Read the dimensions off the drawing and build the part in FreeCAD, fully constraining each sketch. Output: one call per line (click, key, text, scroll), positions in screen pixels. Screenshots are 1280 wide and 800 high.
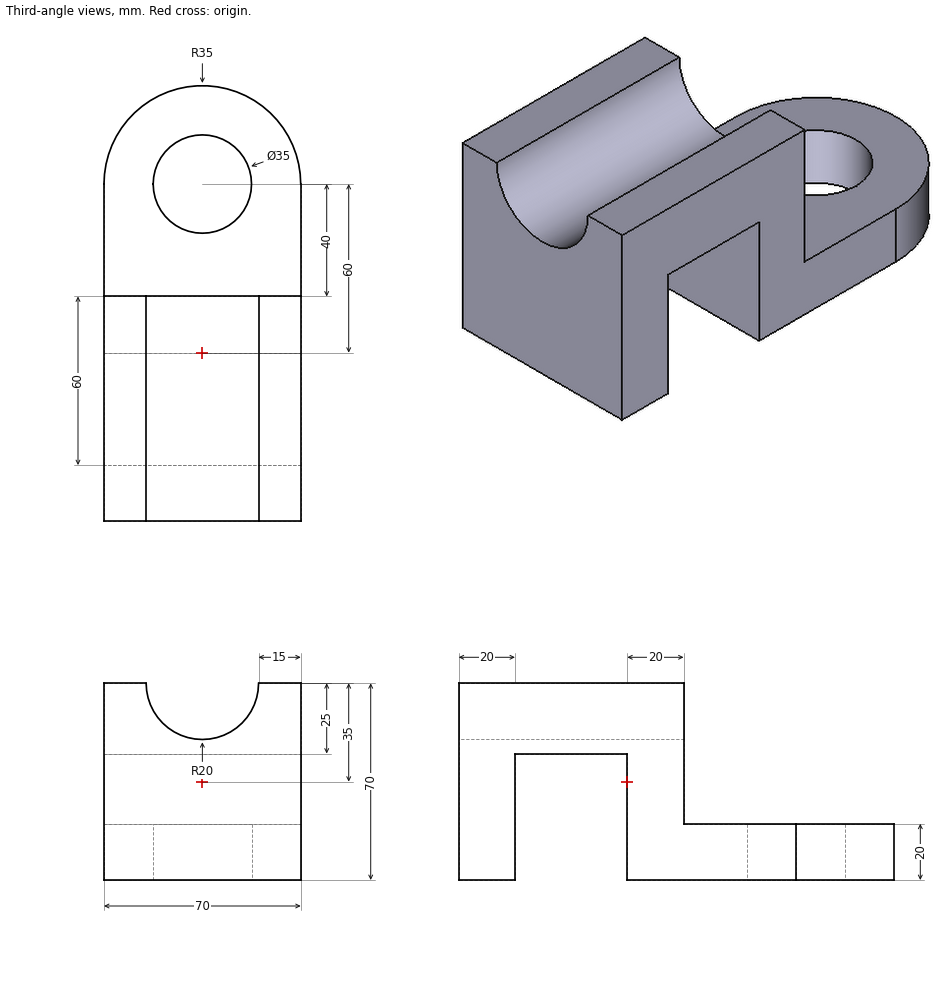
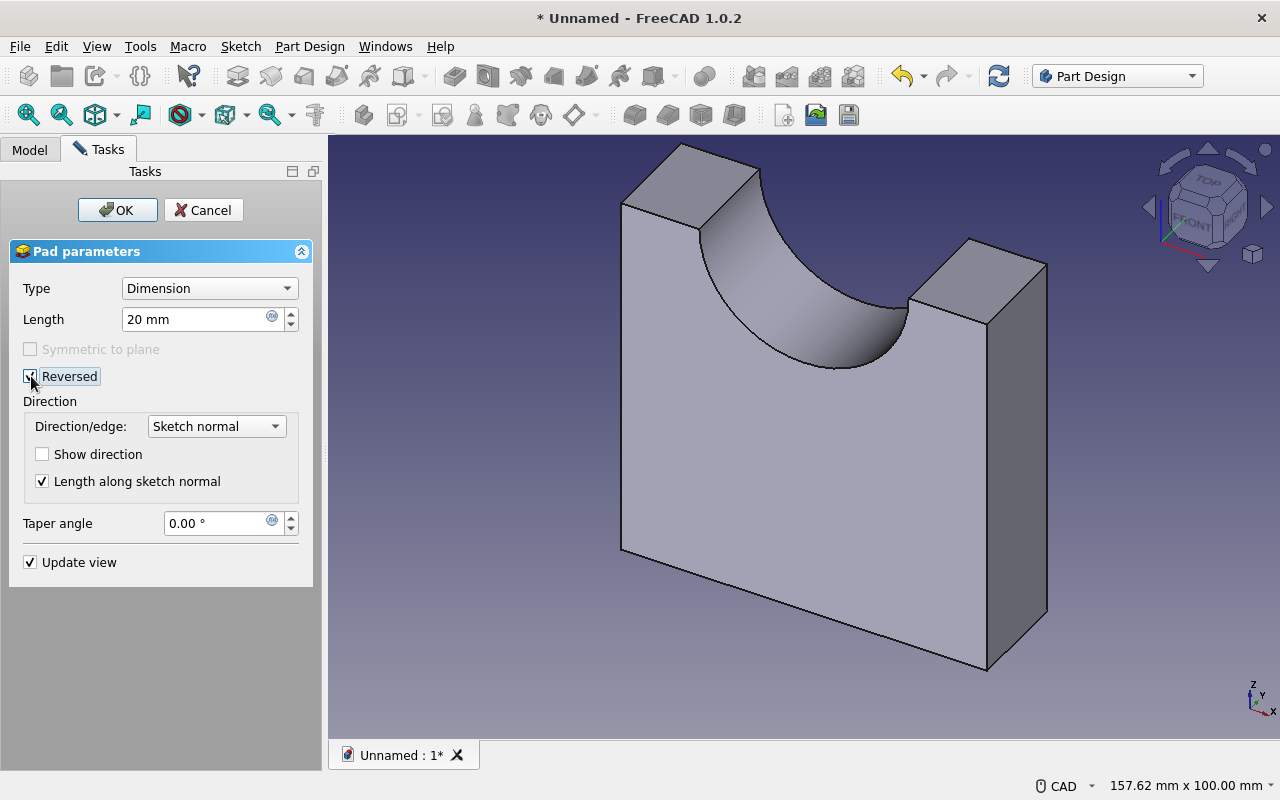
click(118, 210)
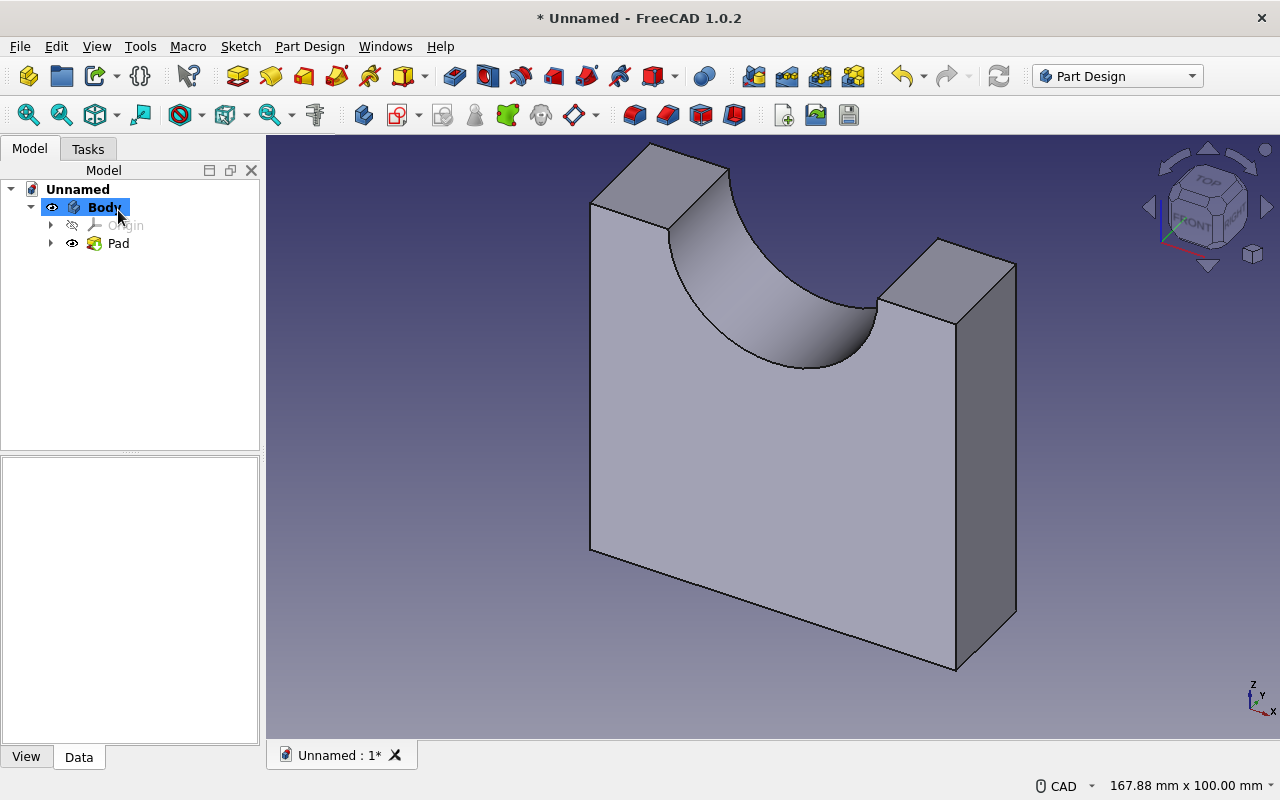
click(51, 225)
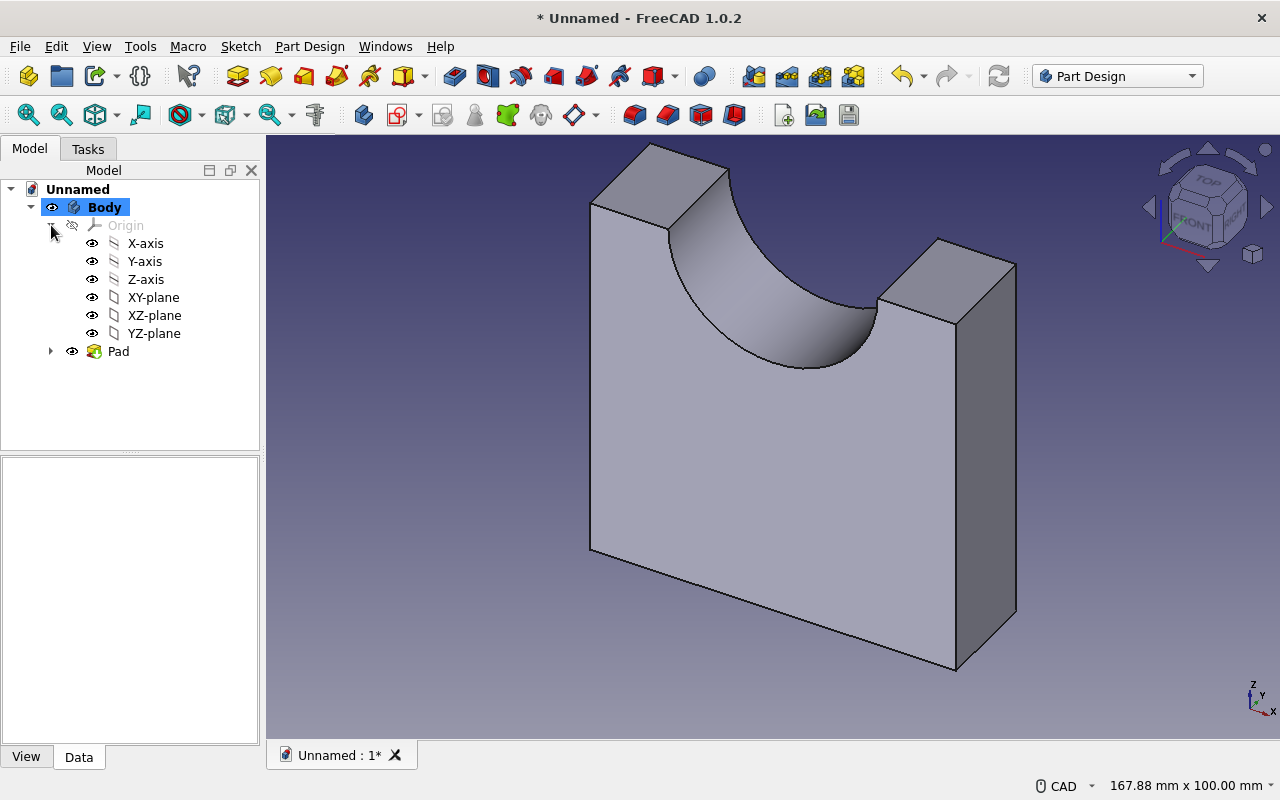
click(137, 315)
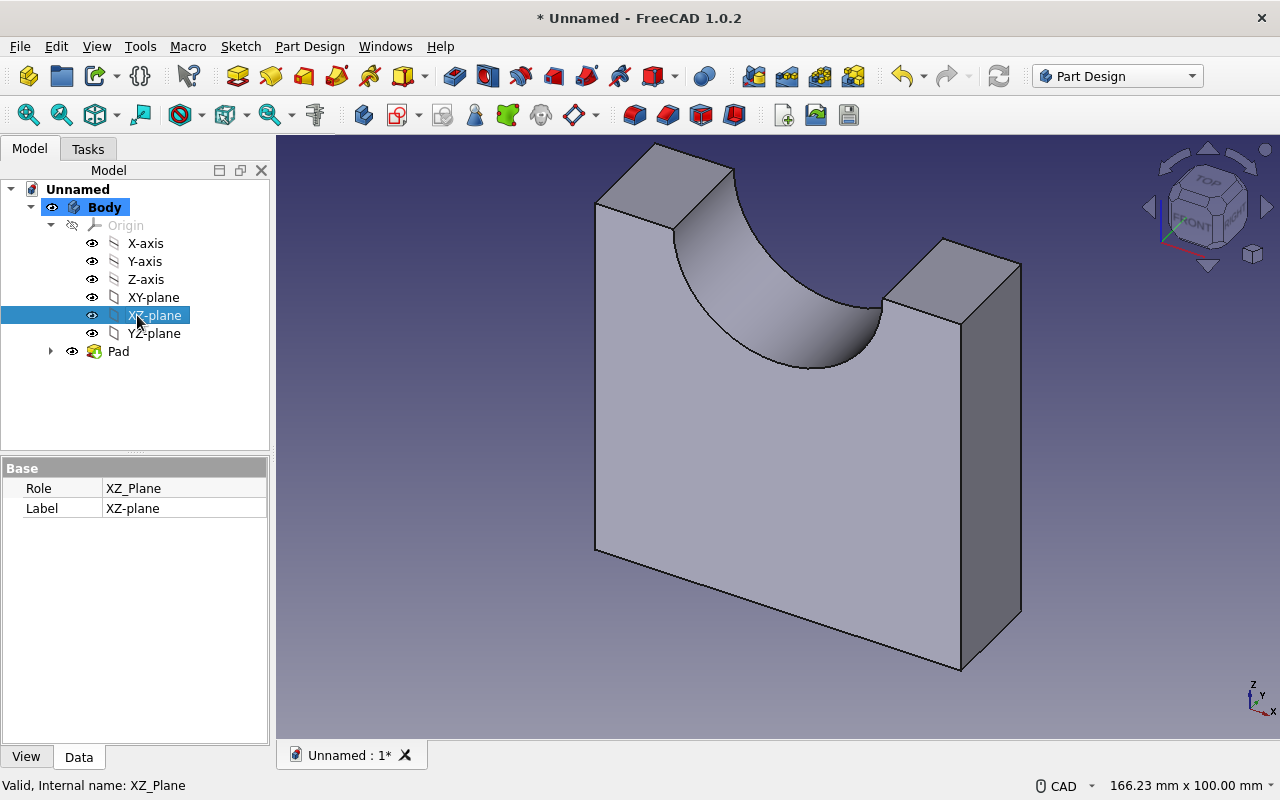
click(574, 116)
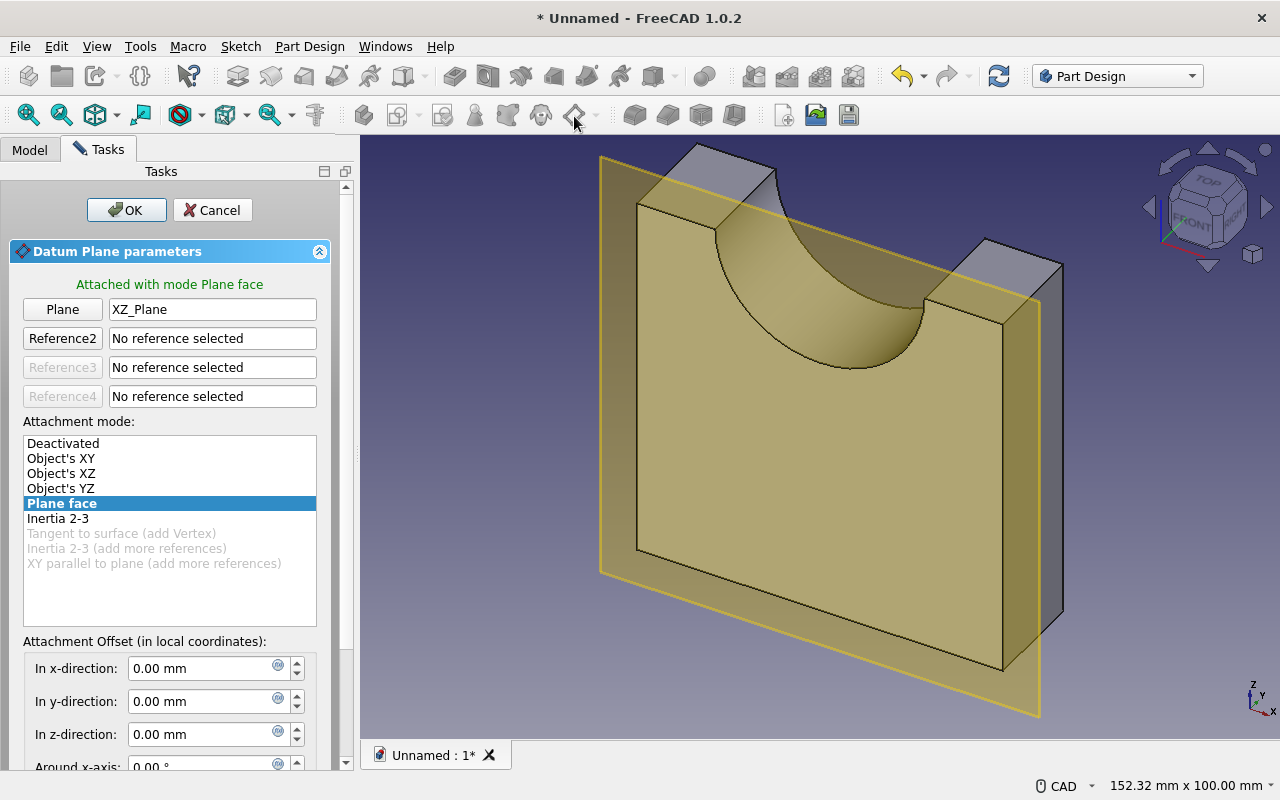
triple_click(210, 734)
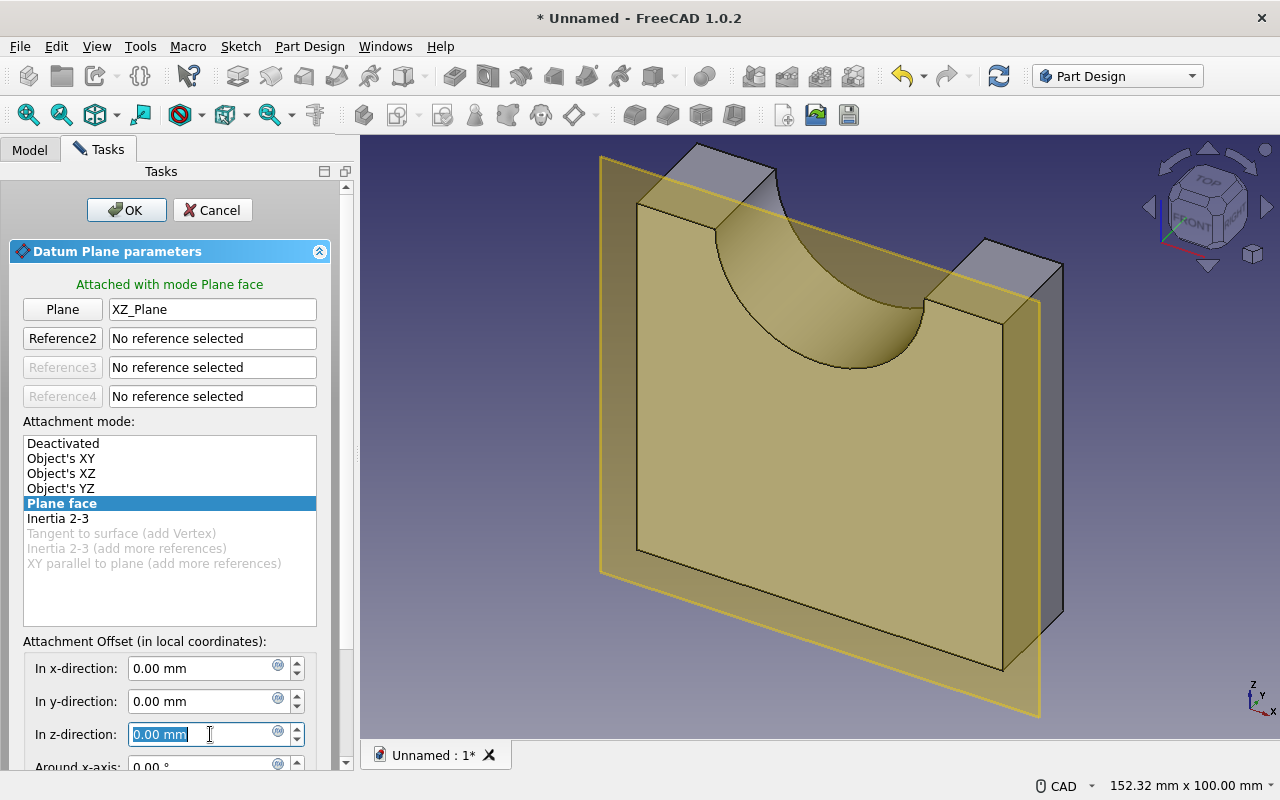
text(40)
key(Tab)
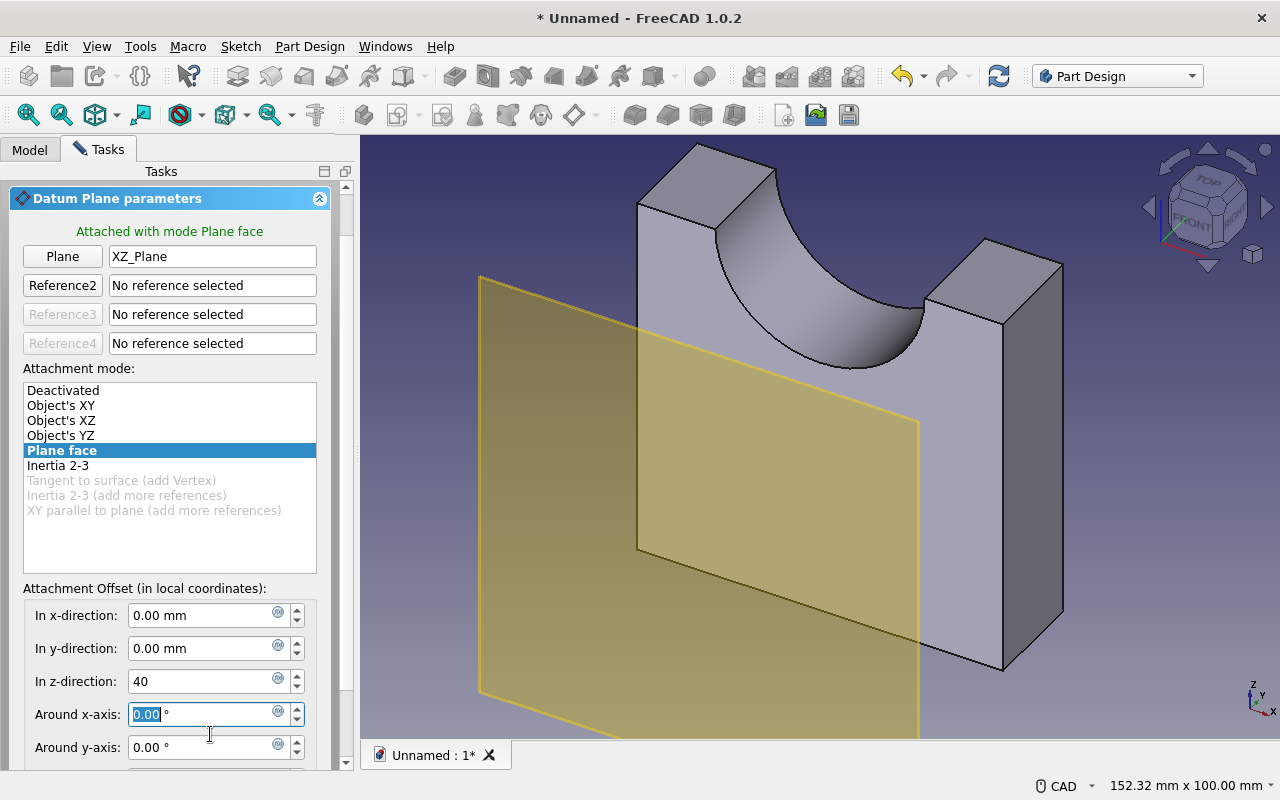
scroll(346, 476, up, 2)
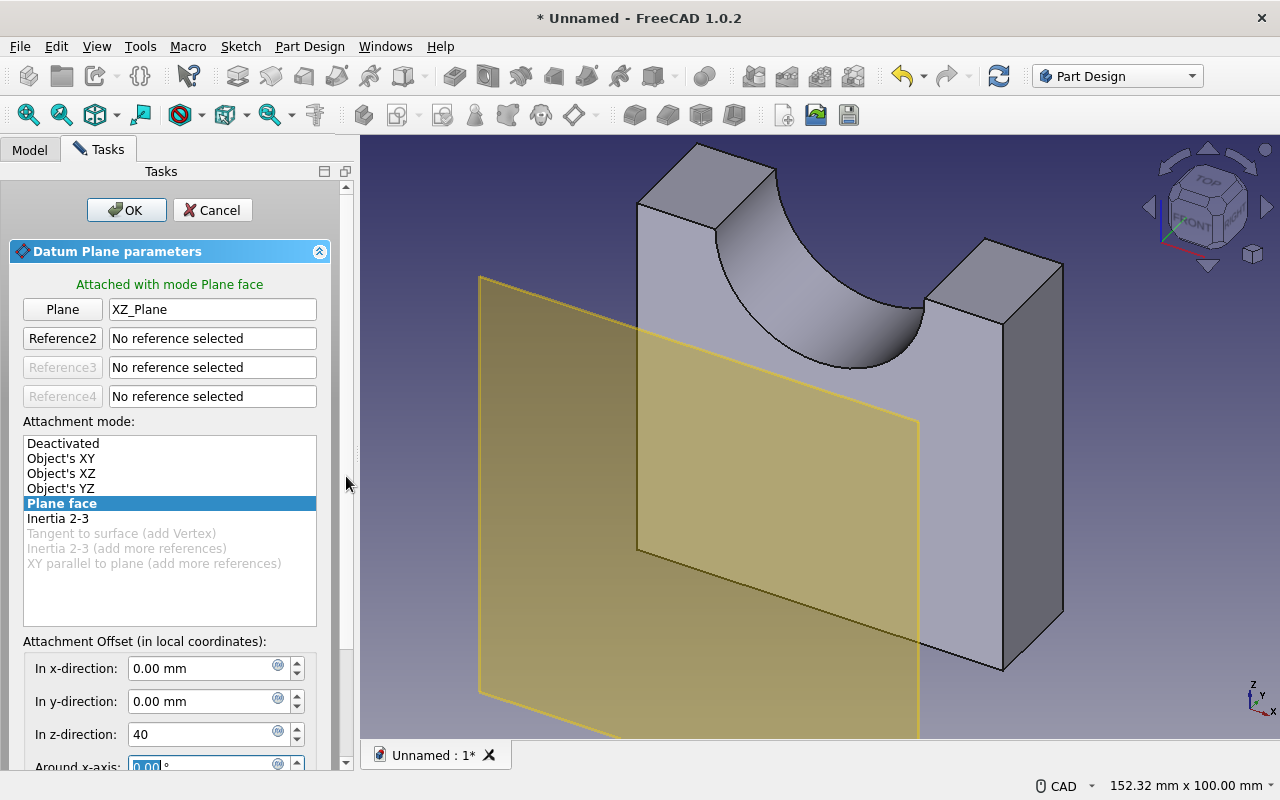
click(127, 210)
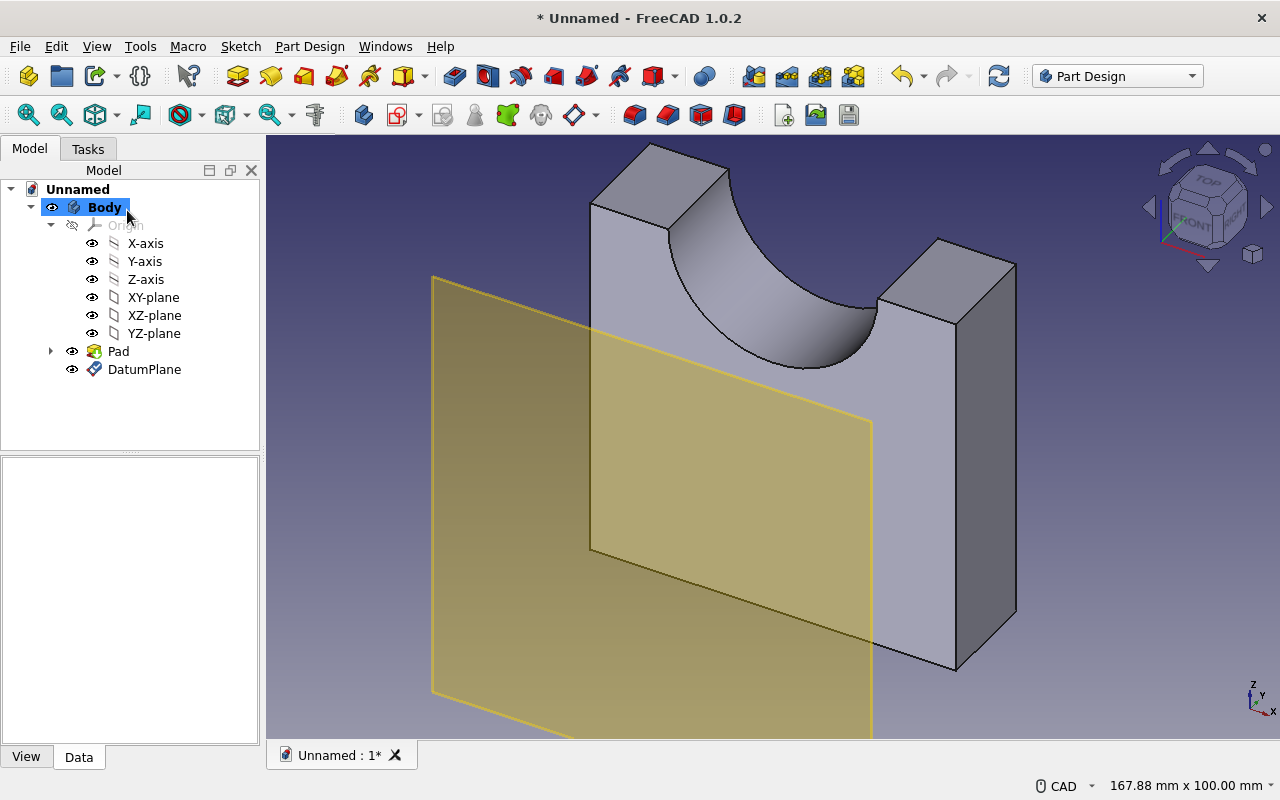
click(117, 369)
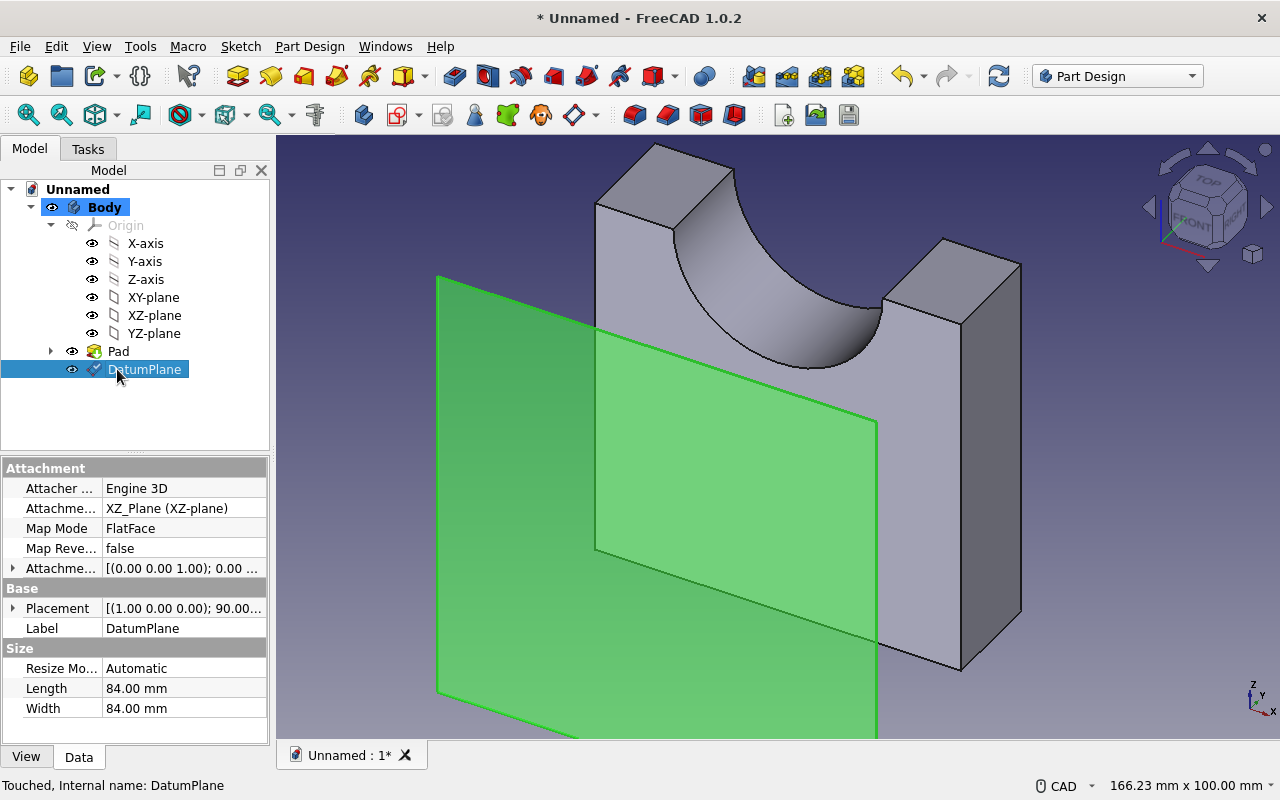
click(396, 116)